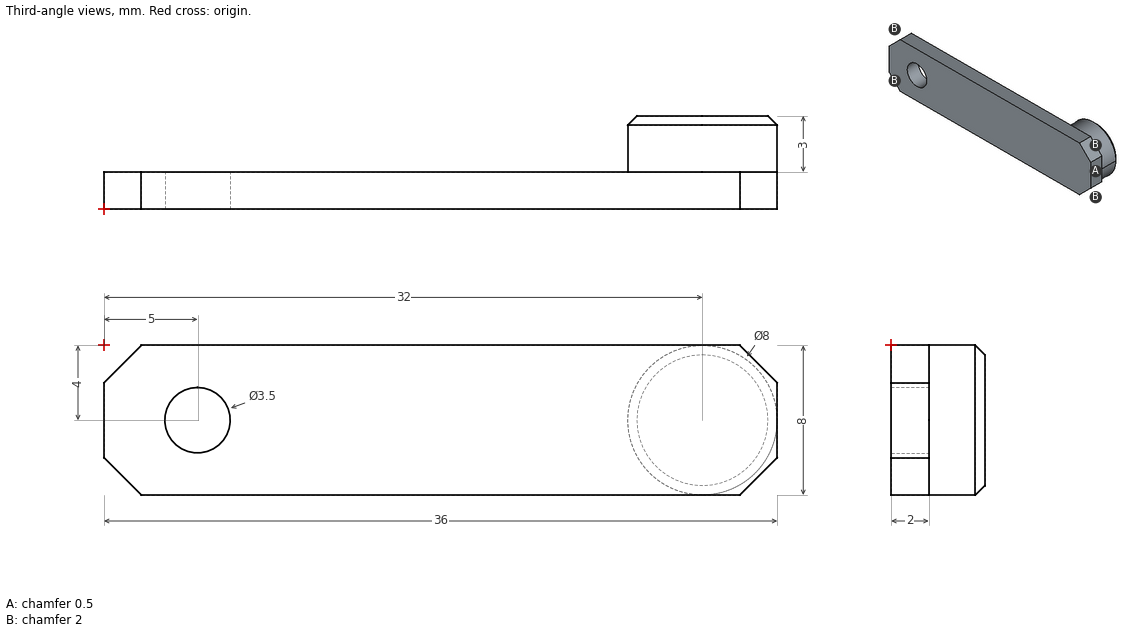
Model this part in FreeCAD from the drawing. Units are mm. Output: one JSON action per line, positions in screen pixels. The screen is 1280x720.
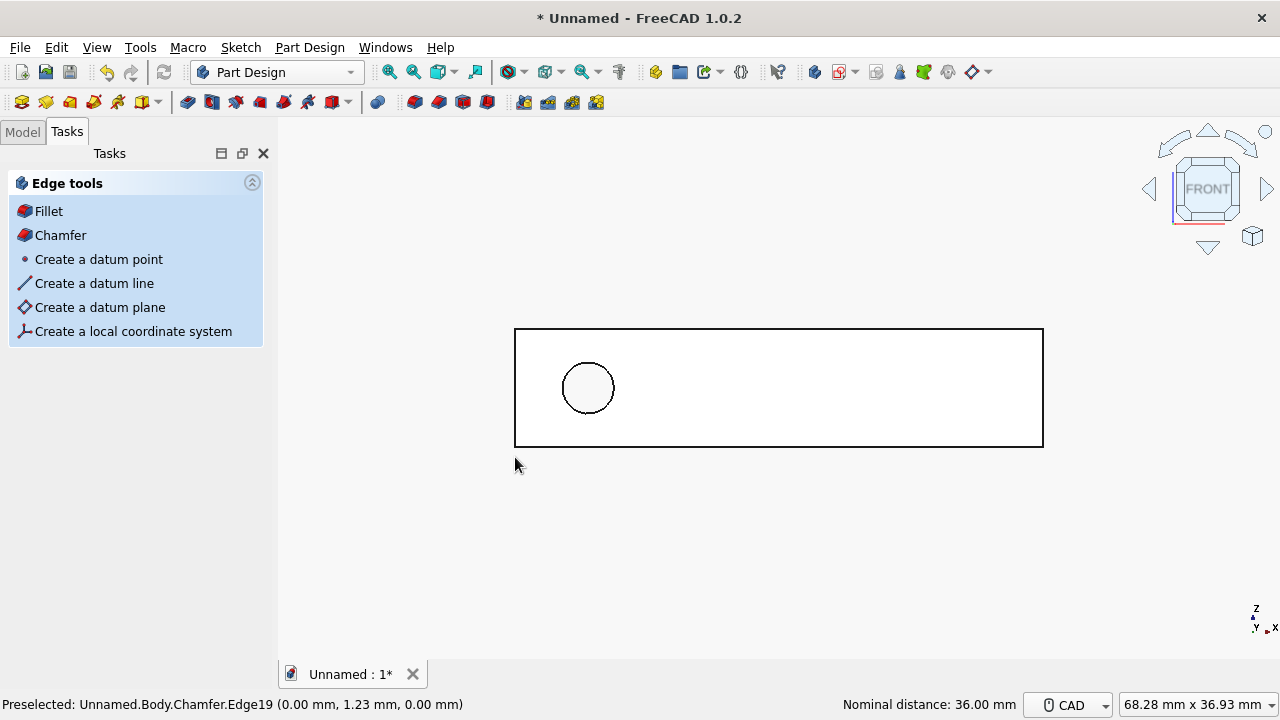
{"action": "key", "text": "3"}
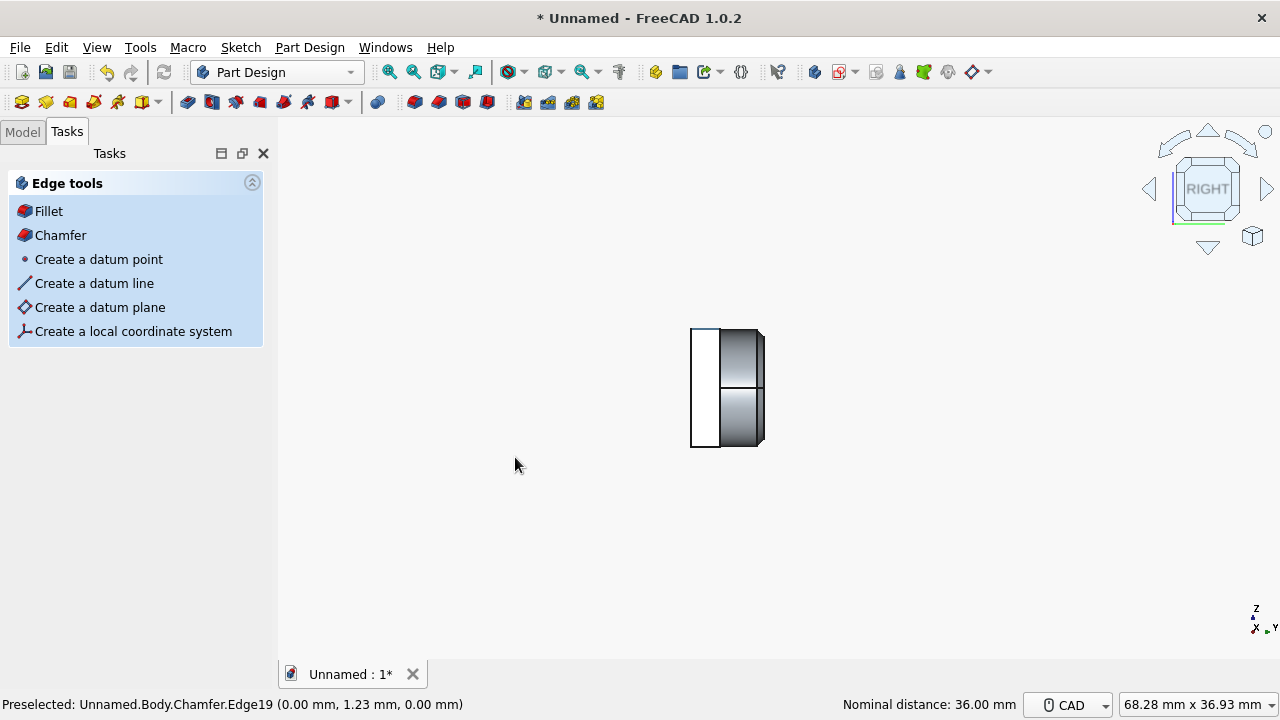
{"action": "key", "text": "v f"}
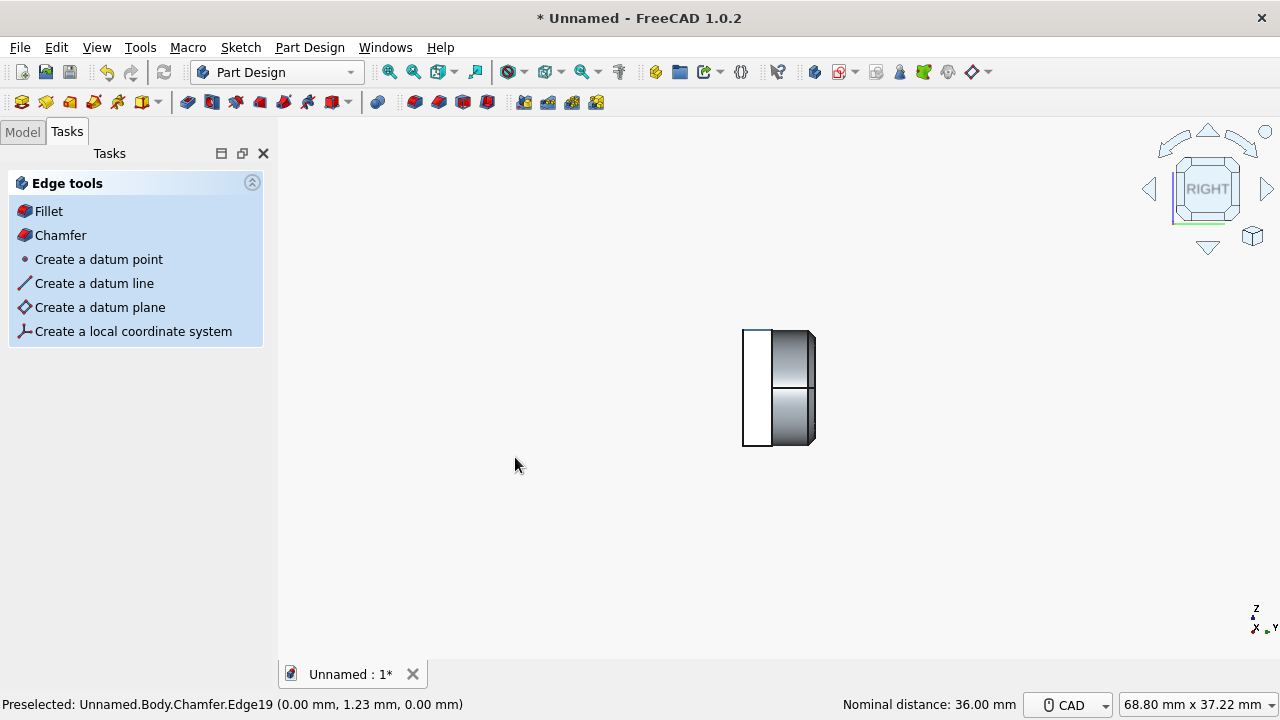
{"action": "left_click", "coordinate": [757, 445], "text": "ctrl"}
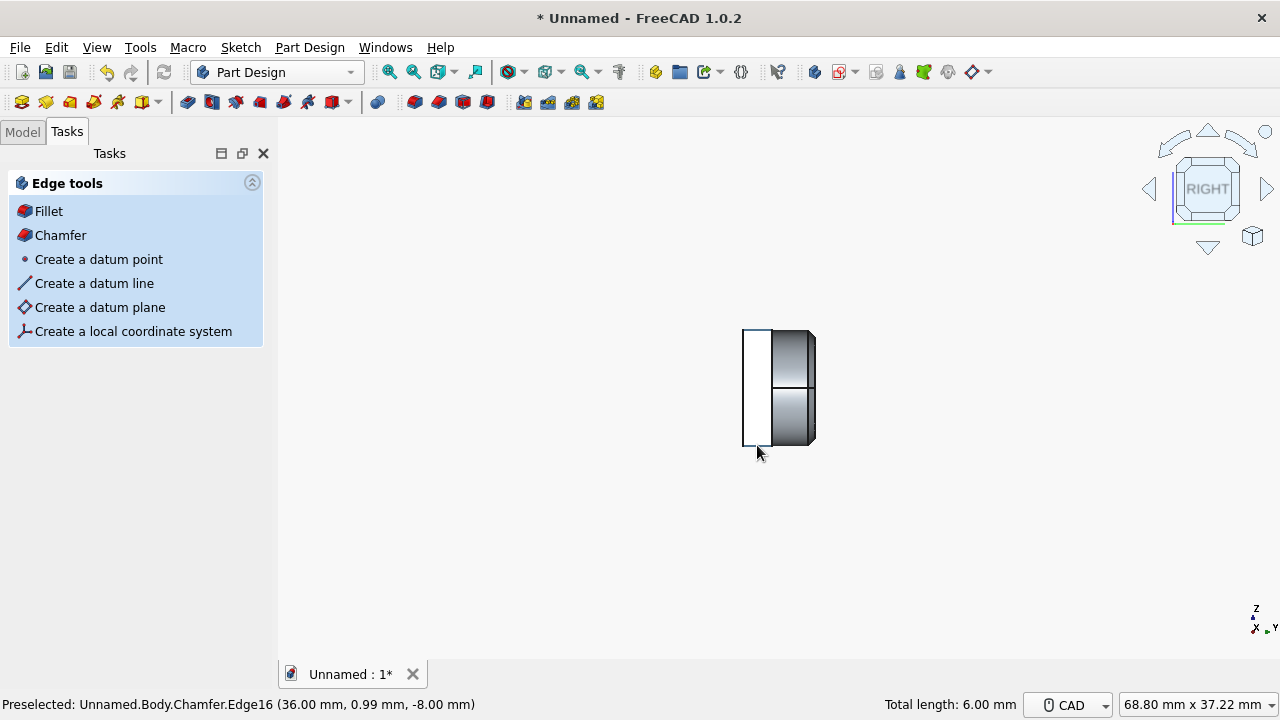
{"action": "key", "text": "5"}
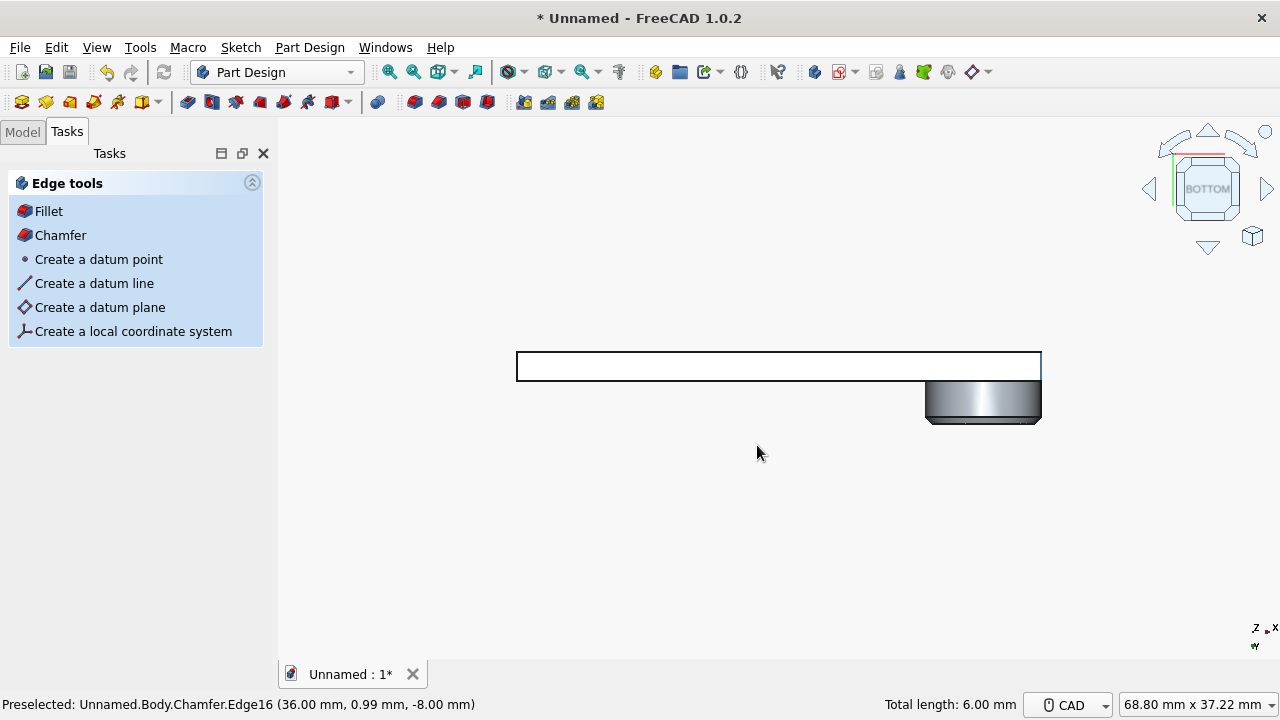
{"action": "left_click", "coordinate": [517, 365], "text": "ctrl"}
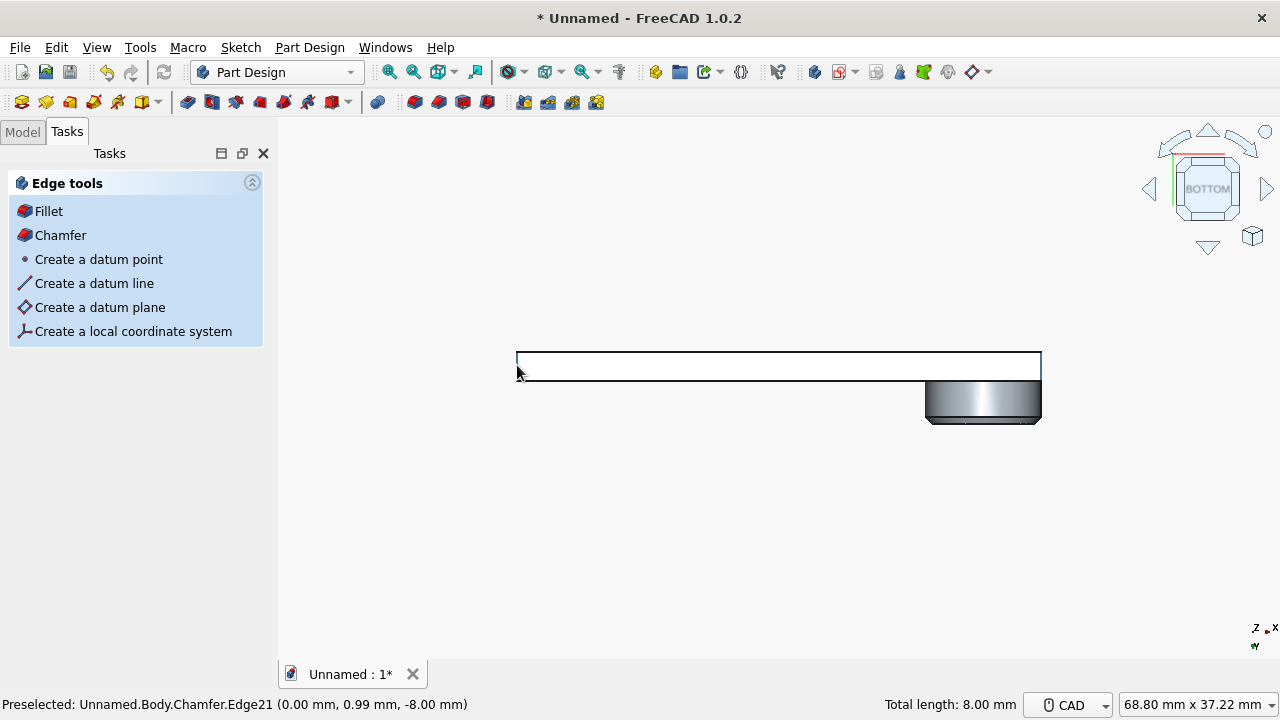
{"action": "left_click", "coordinate": [440, 102]}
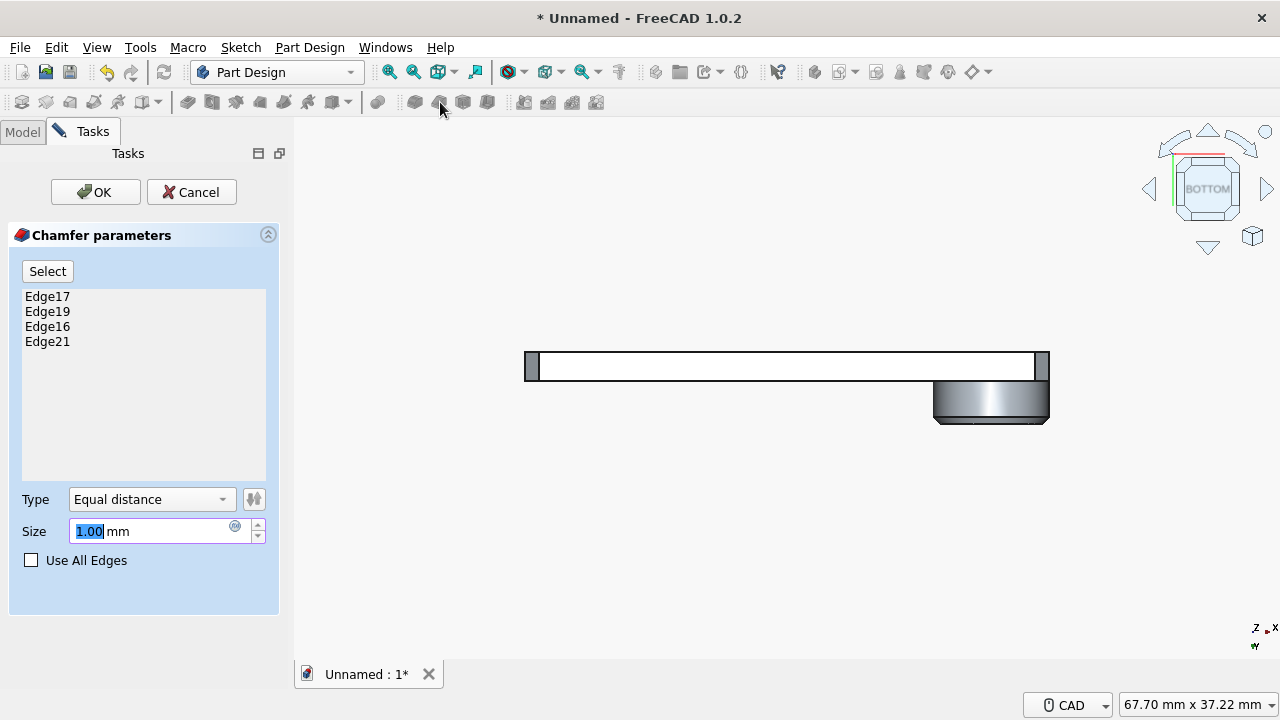
{"action": "type", "text": "2"}
{"action": "key", "text": "Tab"}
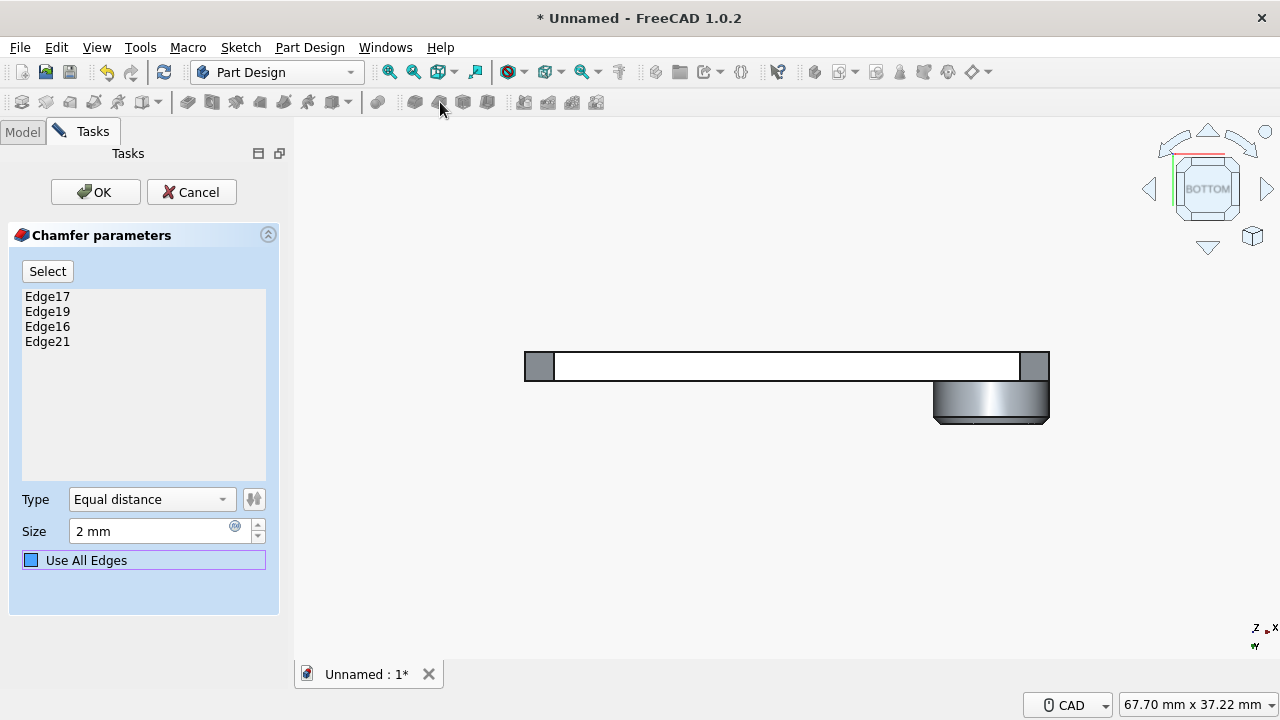
{"action": "left_click", "coordinate": [96, 192]}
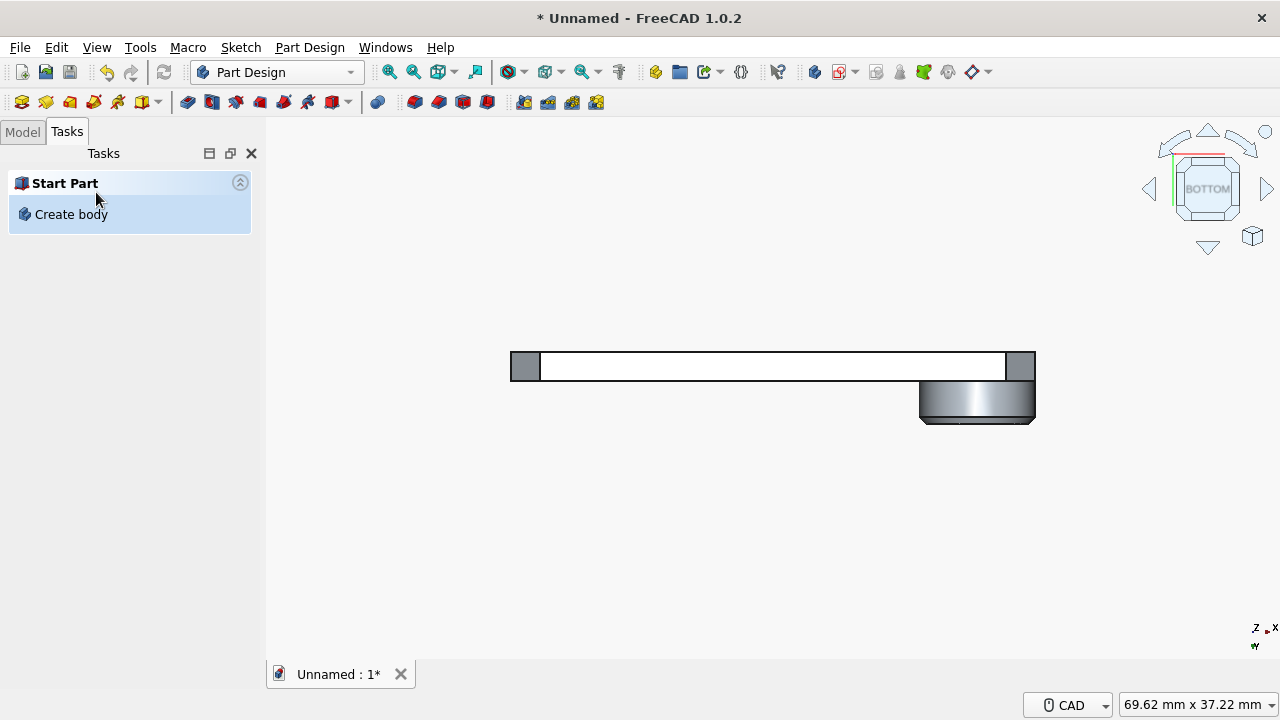
{"action": "key", "text": "0"}